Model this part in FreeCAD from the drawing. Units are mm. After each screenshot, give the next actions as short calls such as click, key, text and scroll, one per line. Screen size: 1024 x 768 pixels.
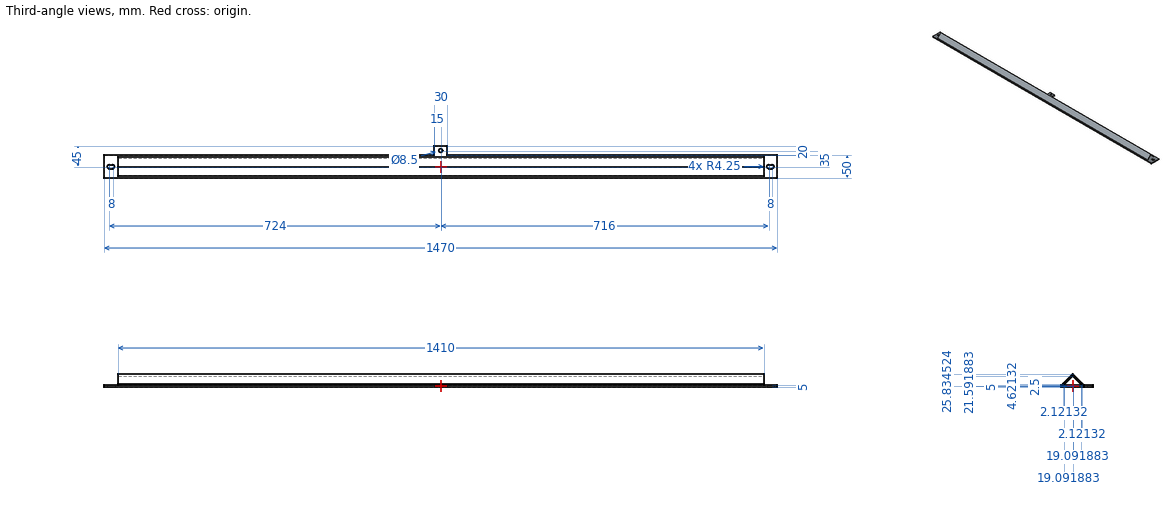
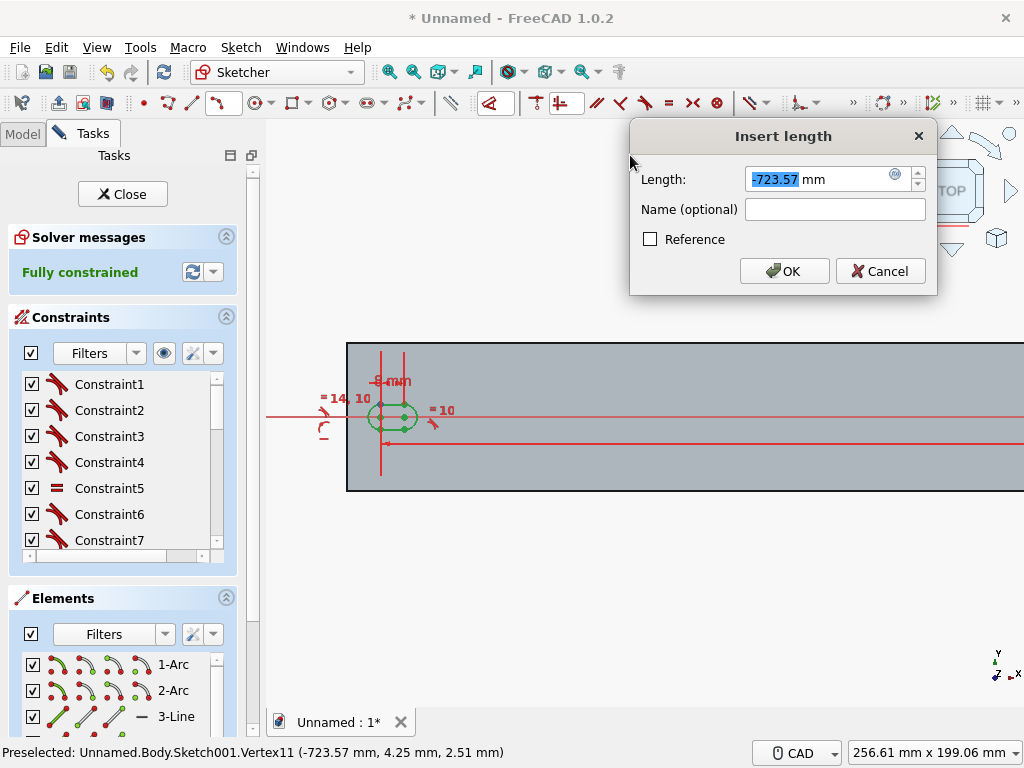
text(-724)
key(Return)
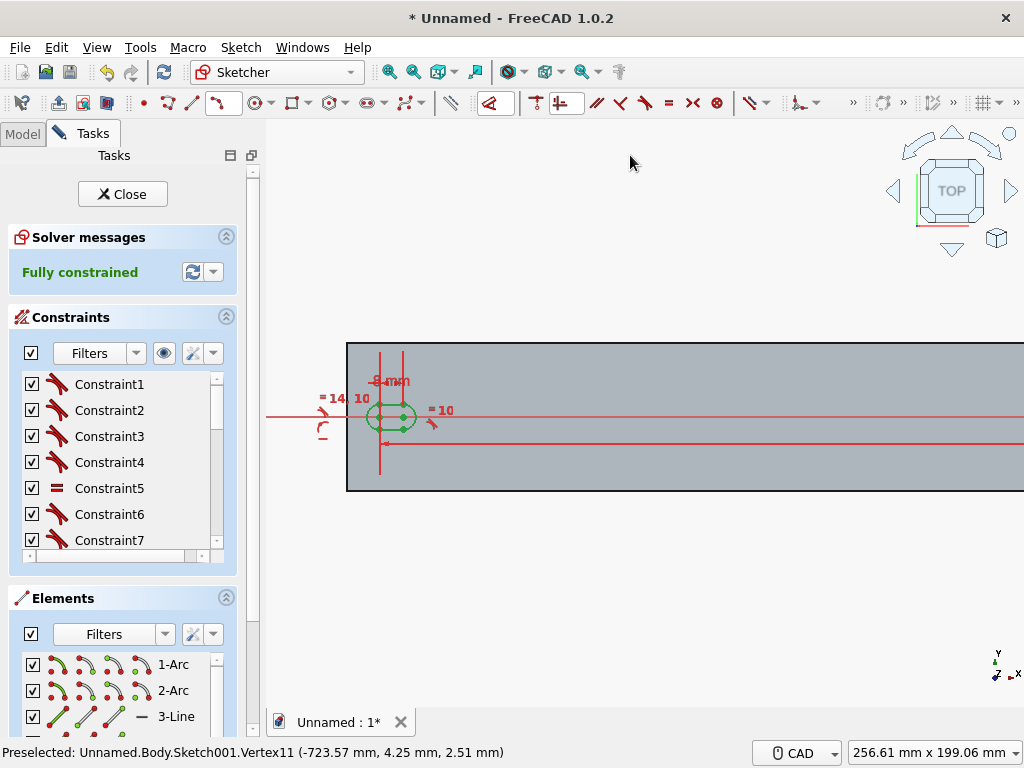
click(123, 194)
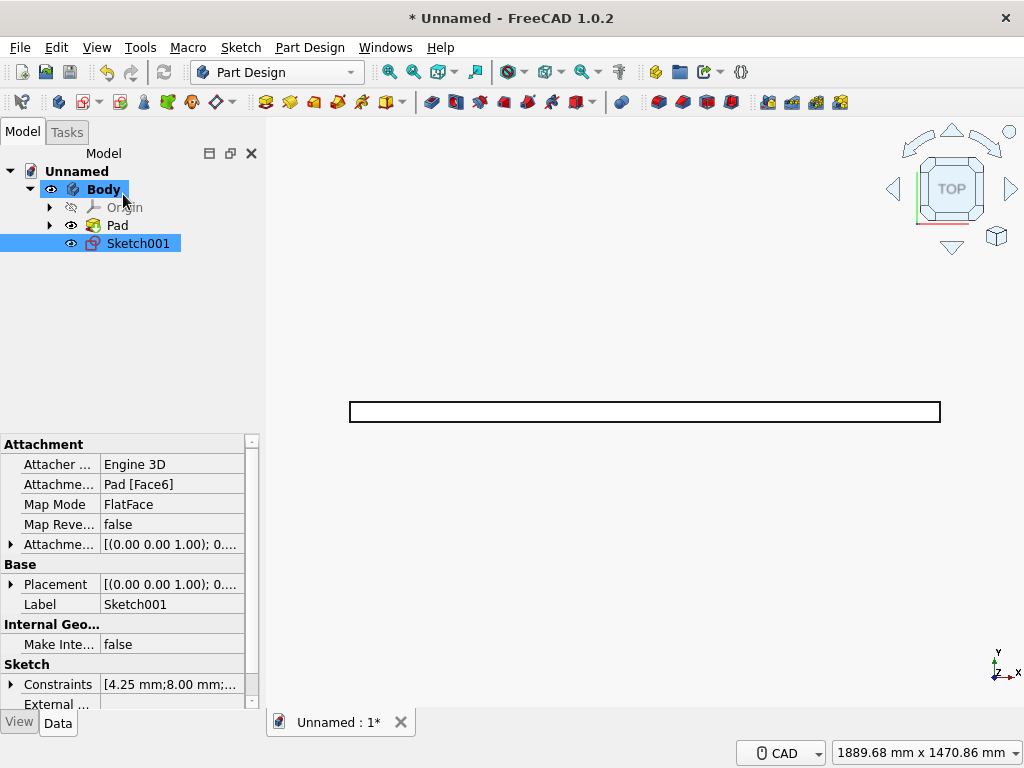
click(432, 102)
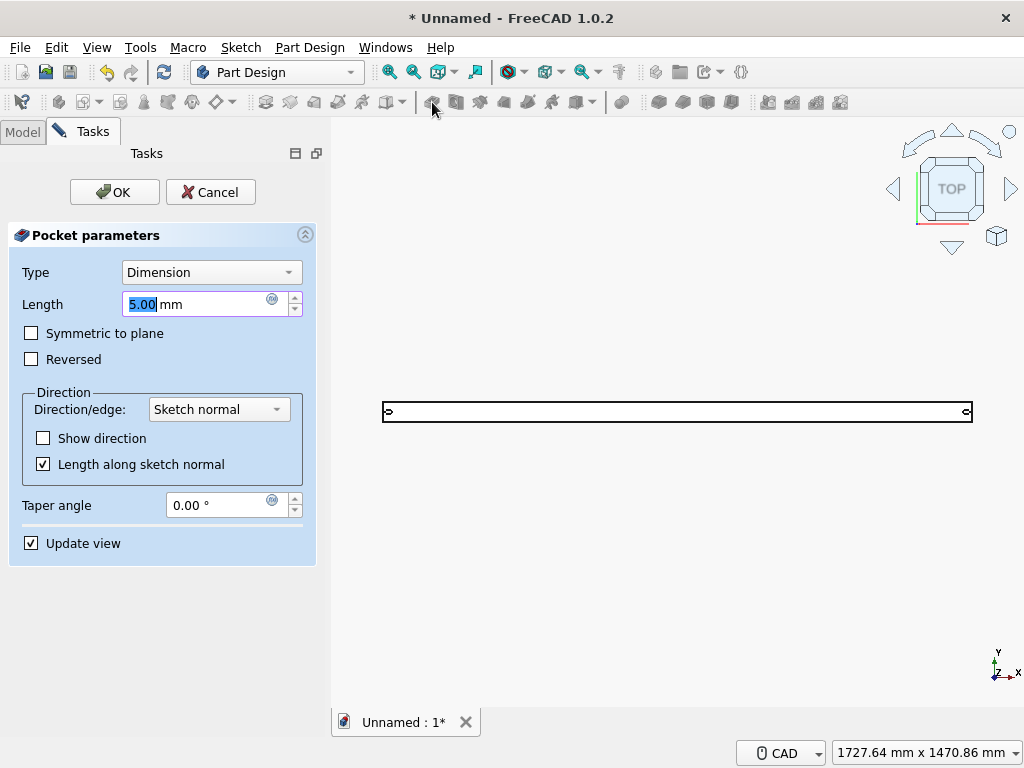
text(5)
key(Tab)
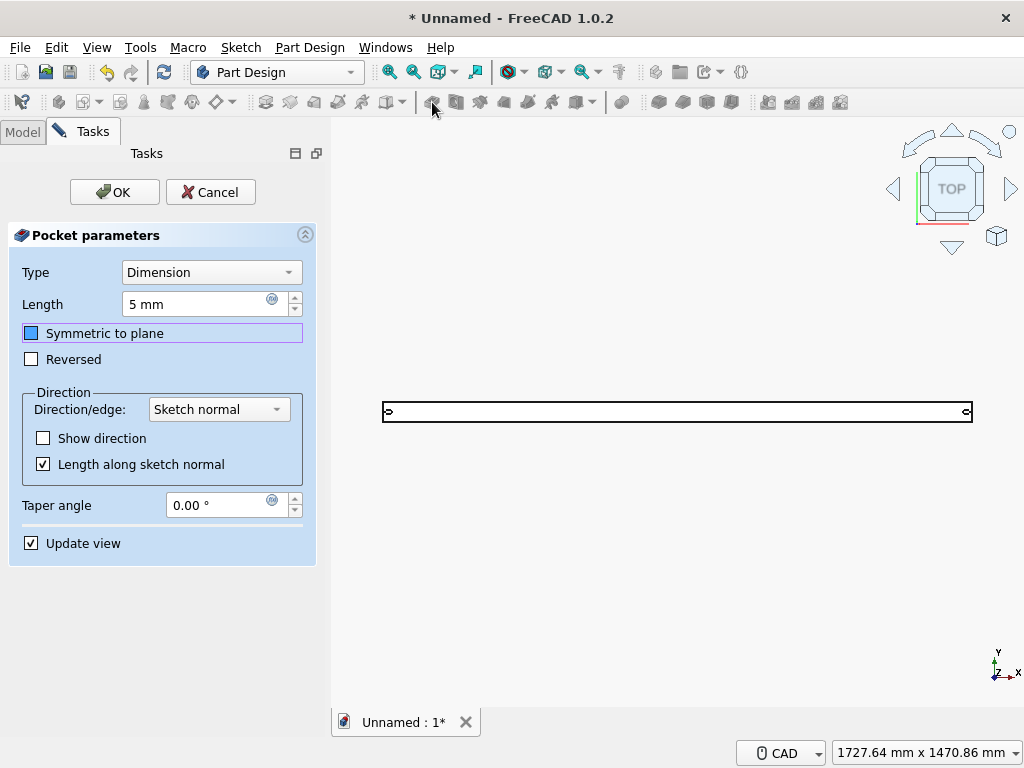
click(115, 192)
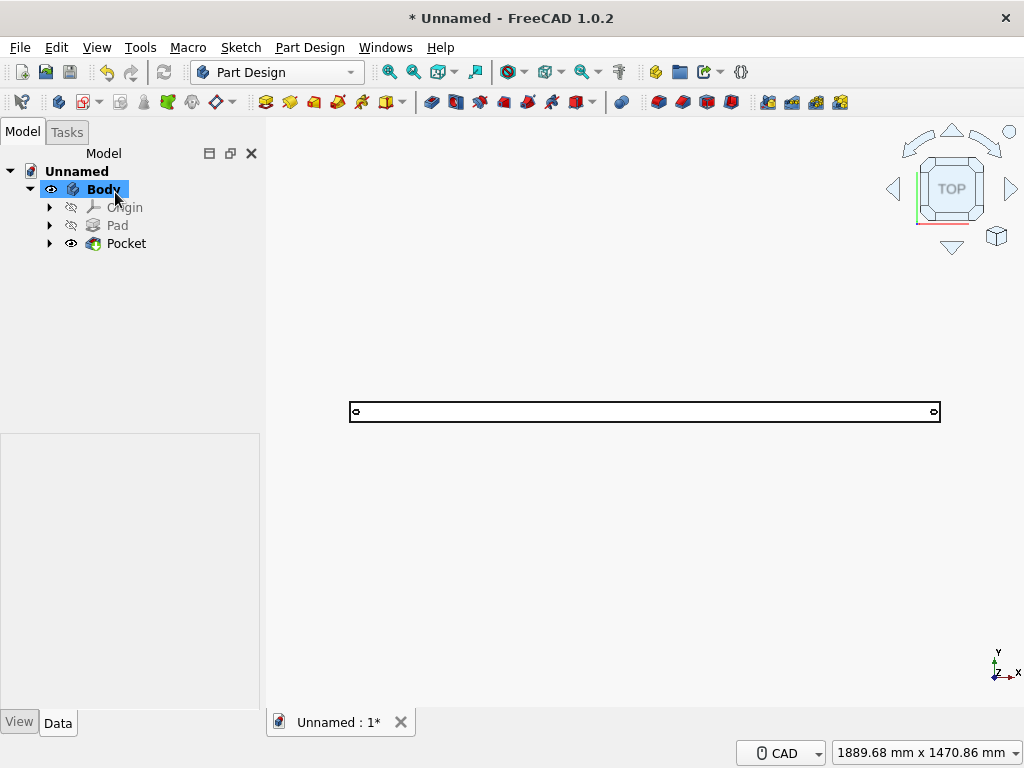
click(898, 411)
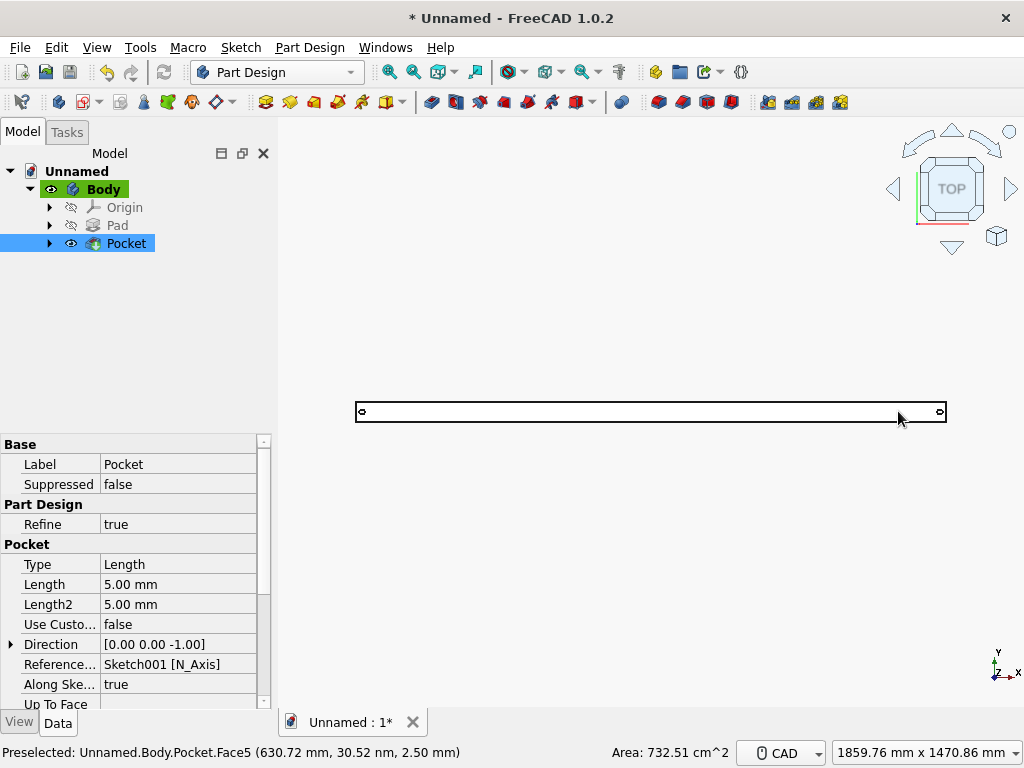
click(84, 102)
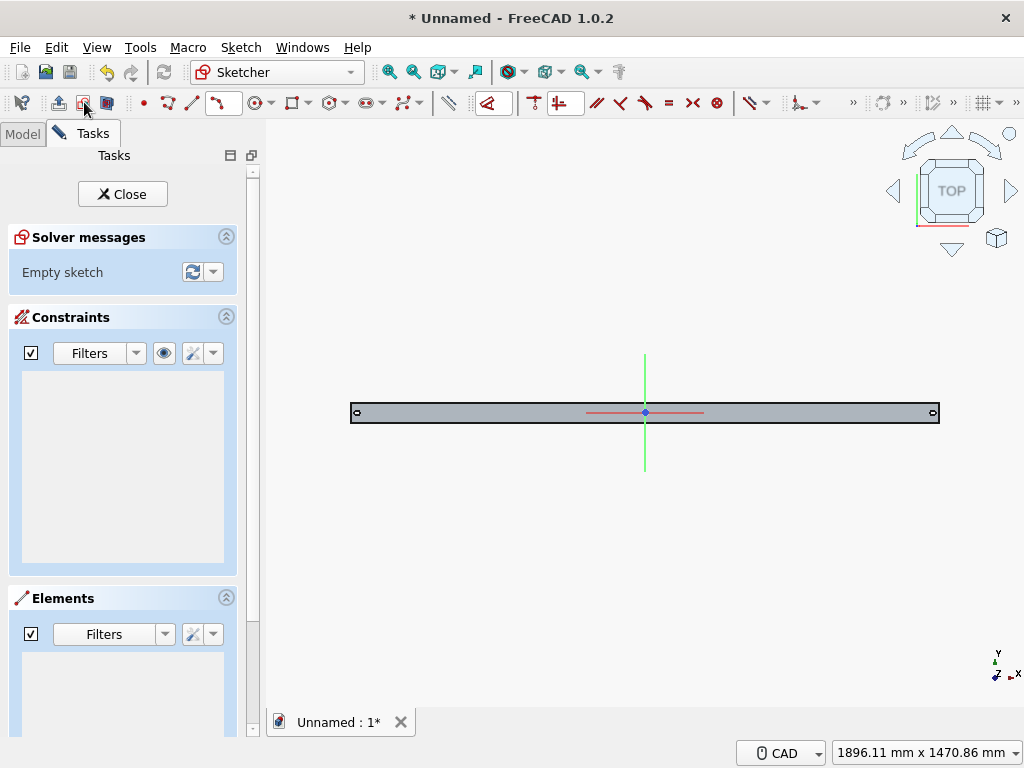
scroll(649, 404, up, 15)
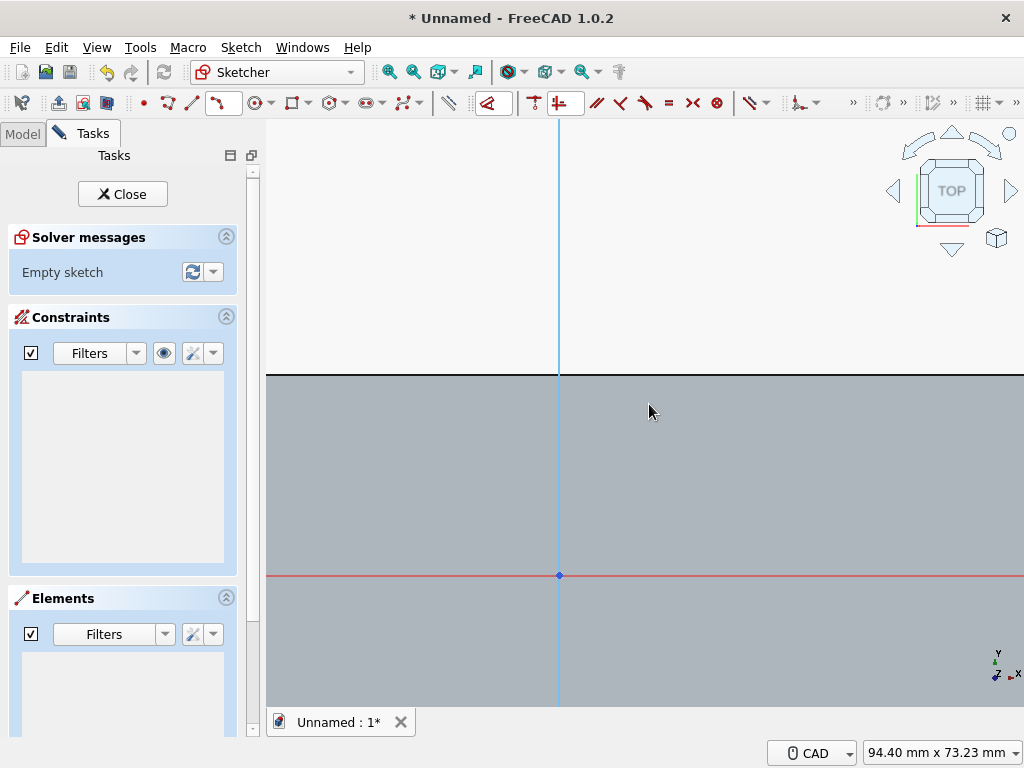
click(292, 104)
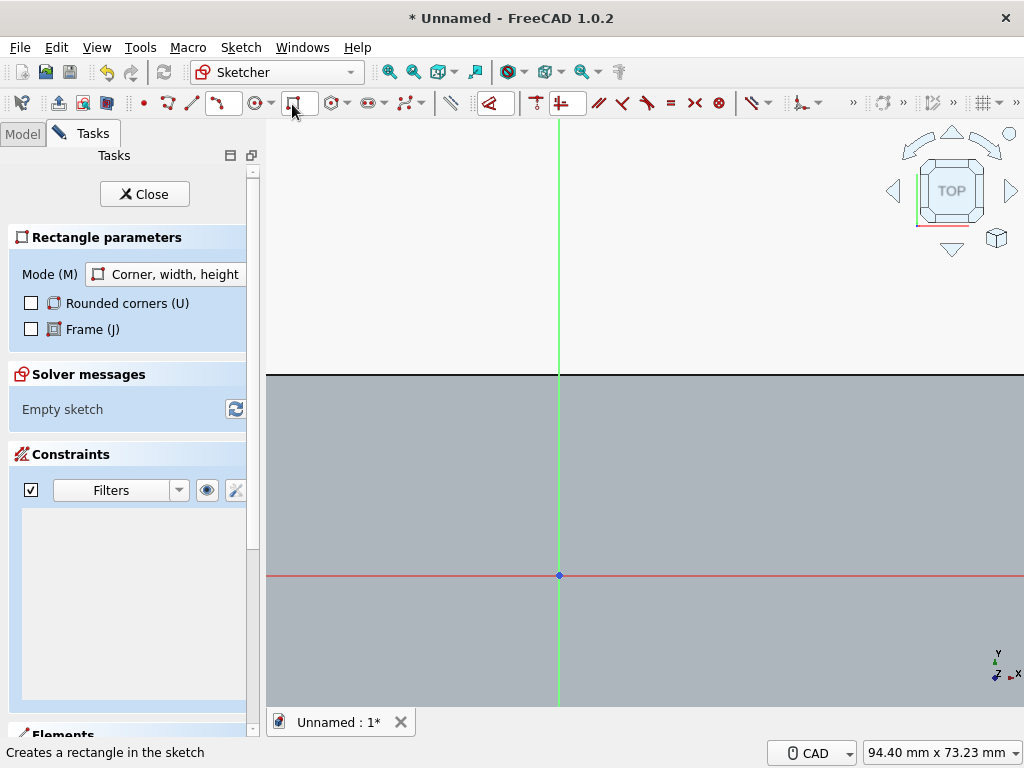
click(439, 214)
move(679, 375)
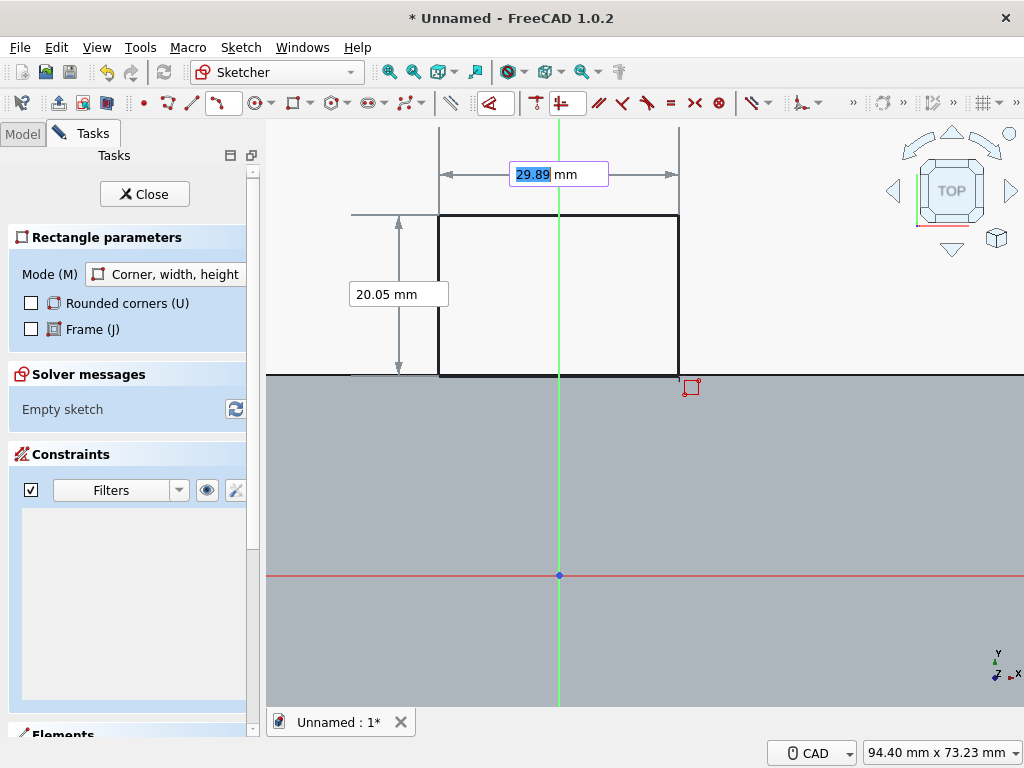
text(30)
key(Tab)
text(20)
key(Return)
key(Escape)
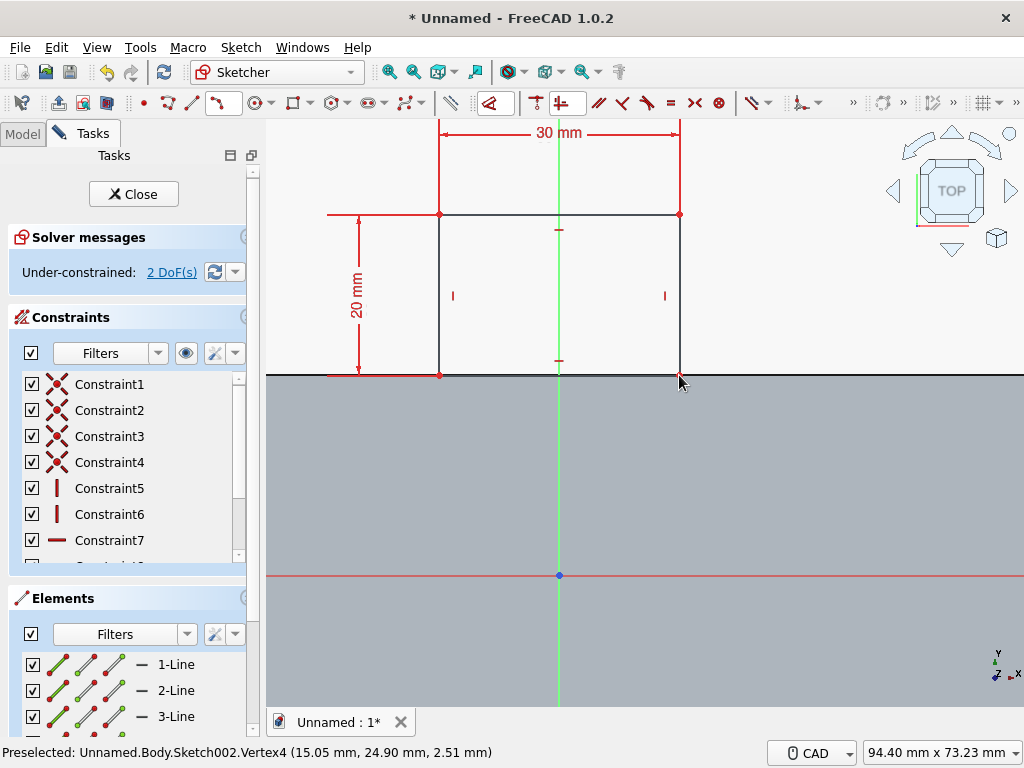
click(439, 215)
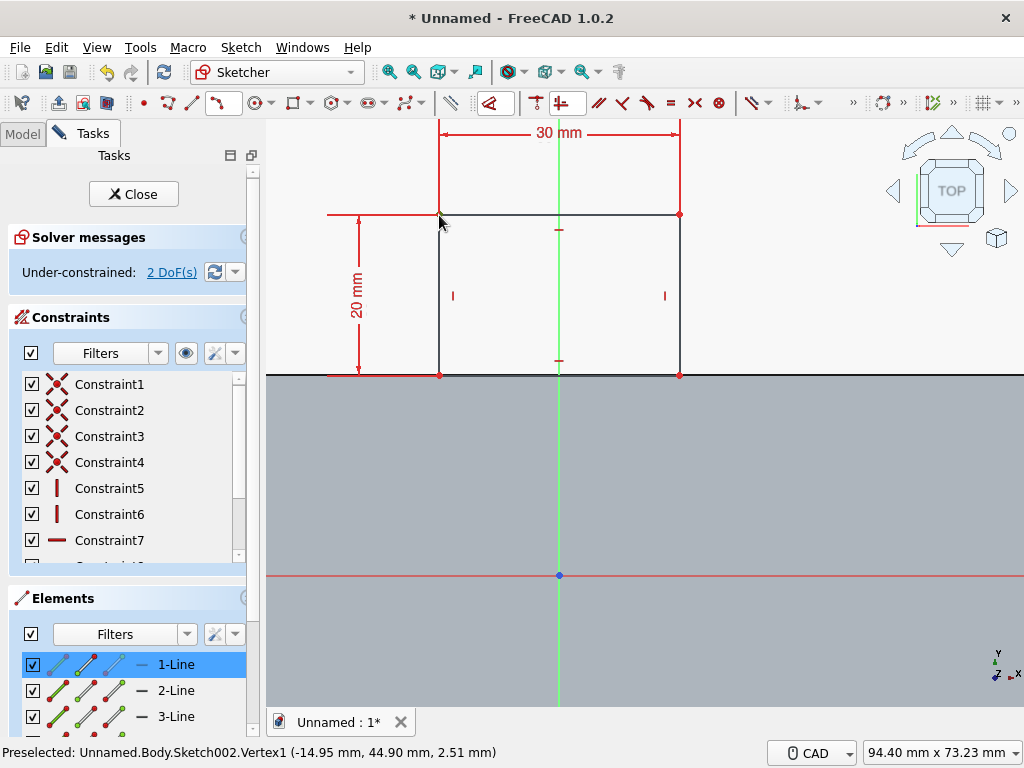
click(508, 104)